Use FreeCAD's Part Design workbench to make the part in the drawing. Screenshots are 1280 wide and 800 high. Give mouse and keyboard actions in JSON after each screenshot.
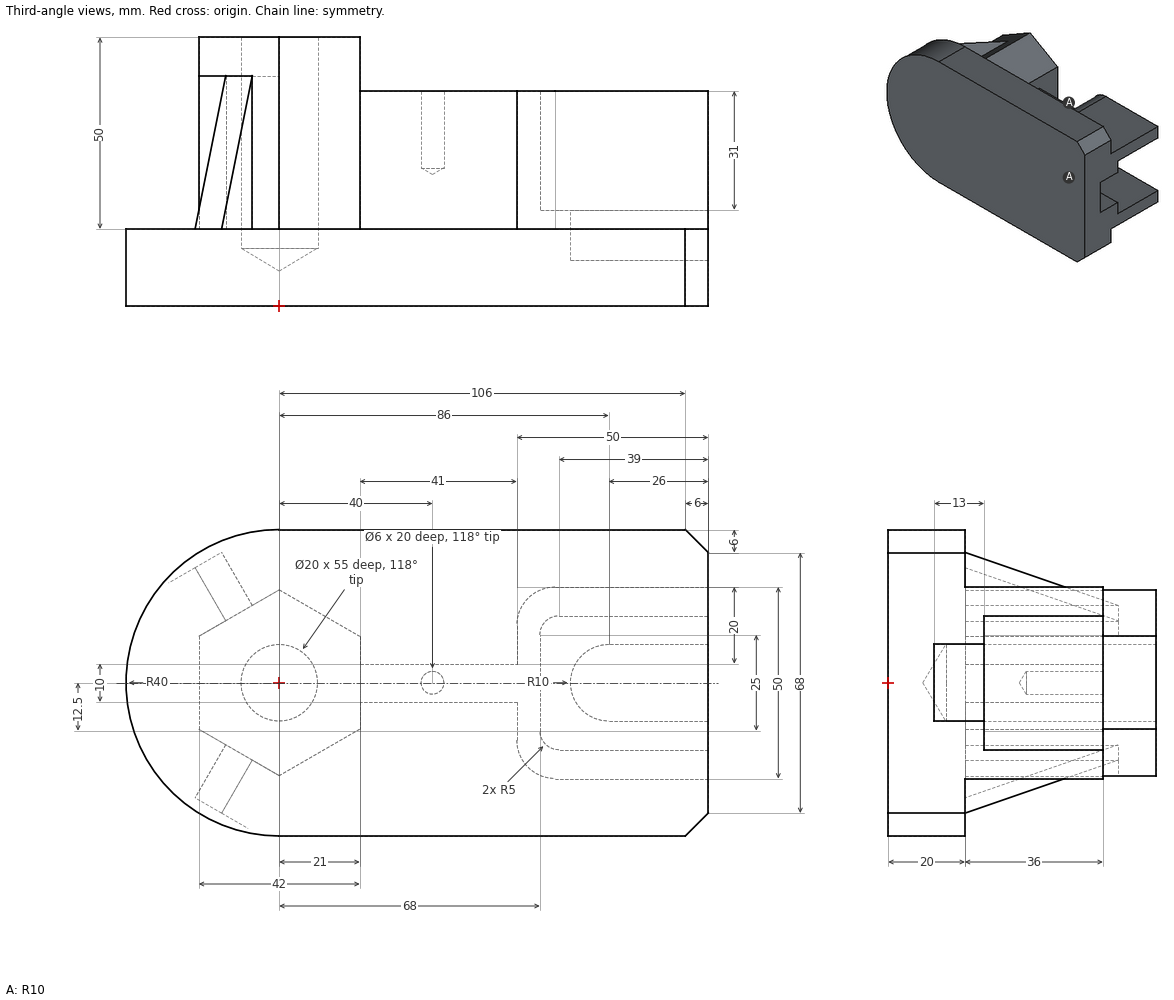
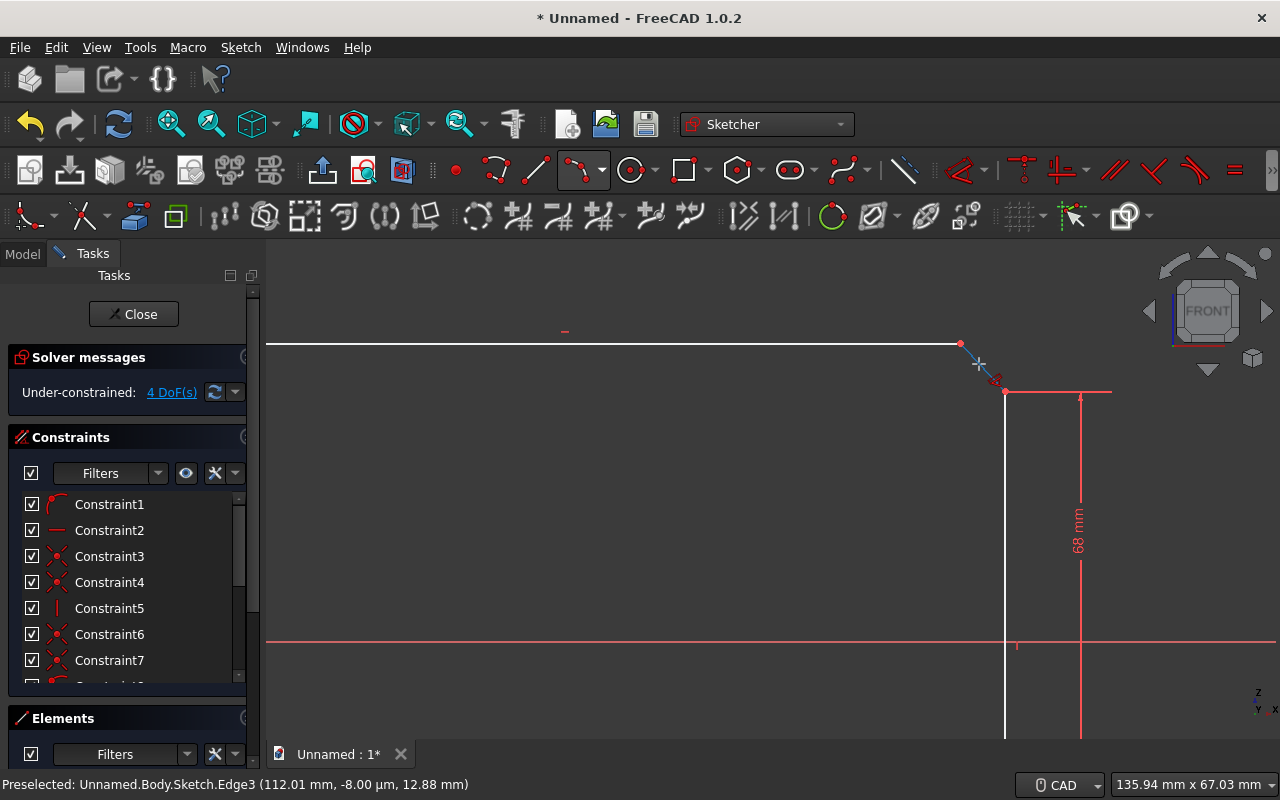
{"action": "left_click", "coordinate": [979, 363]}
{"action": "left_click", "coordinate": [983, 310]}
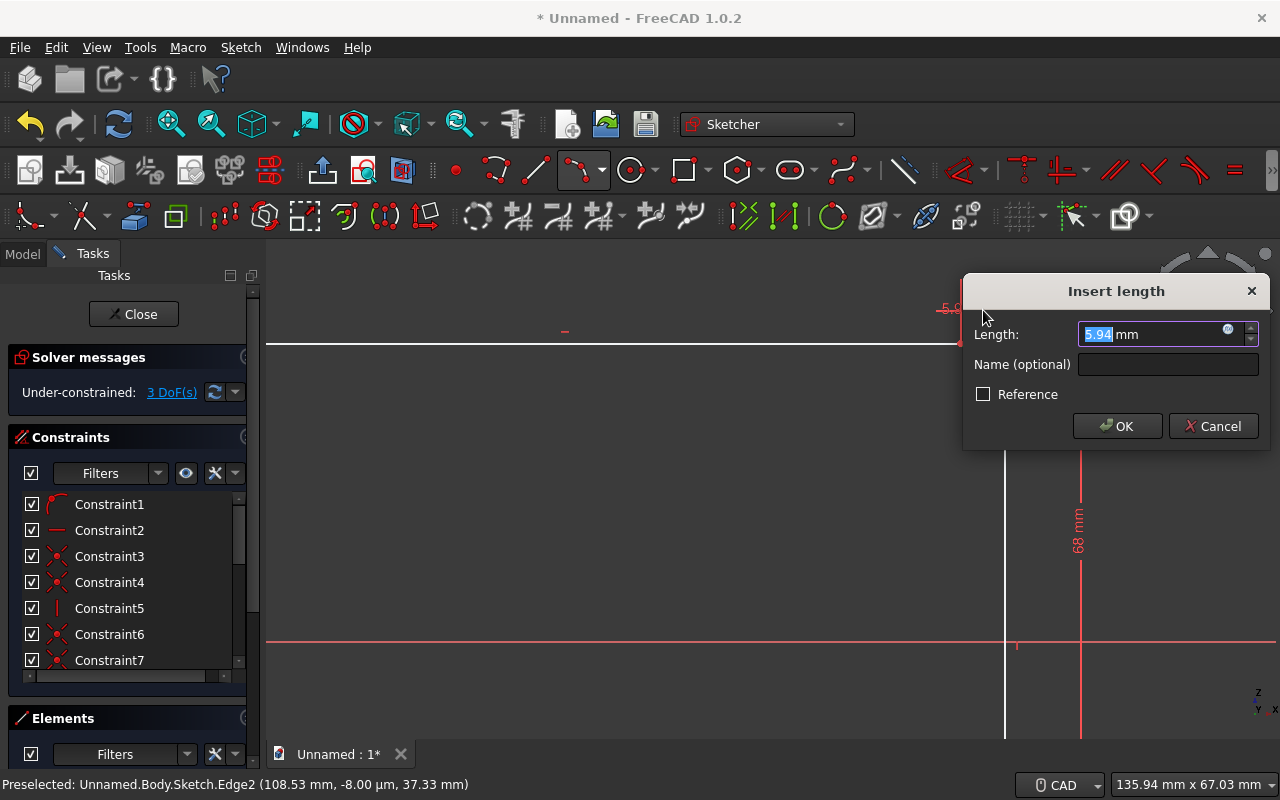
{"action": "type", "text": "6"}
{"action": "key", "text": "Return"}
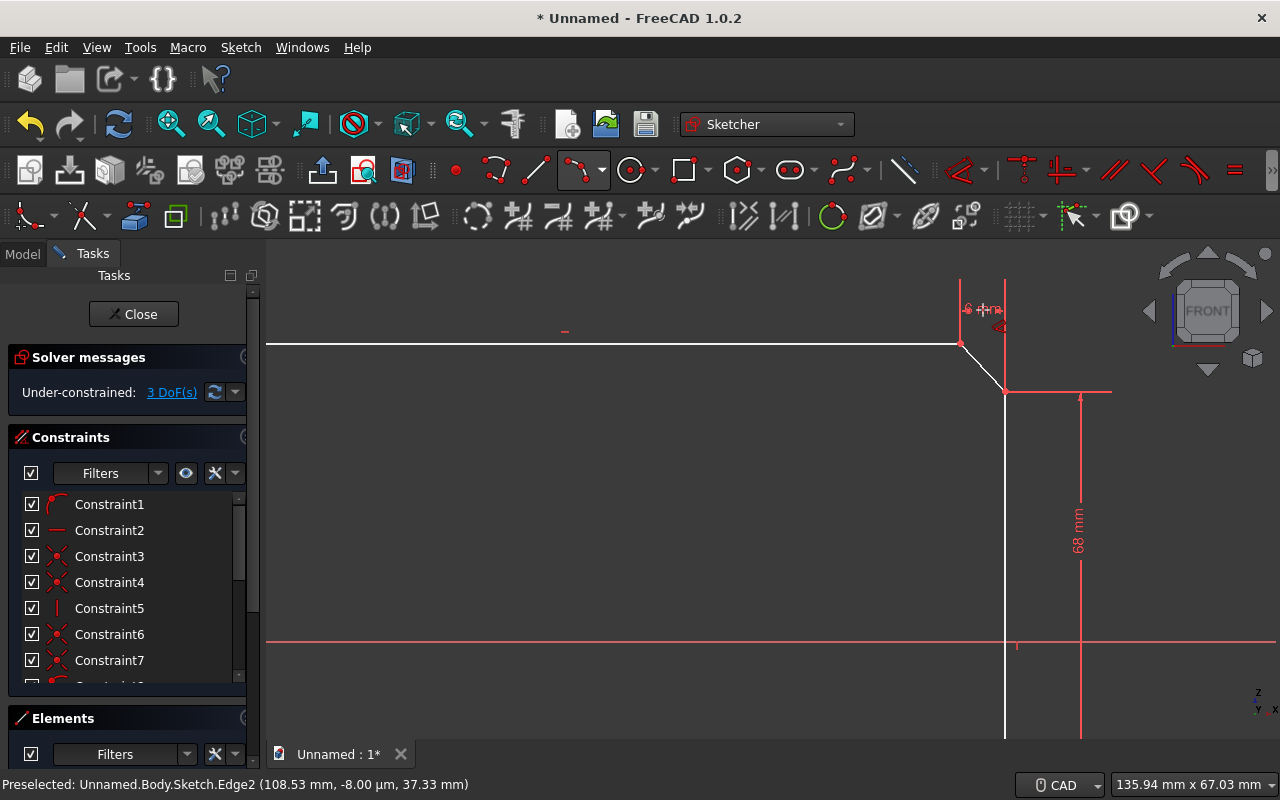
{"action": "left_click", "coordinate": [974, 358]}
{"action": "left_click", "coordinate": [1039, 368]}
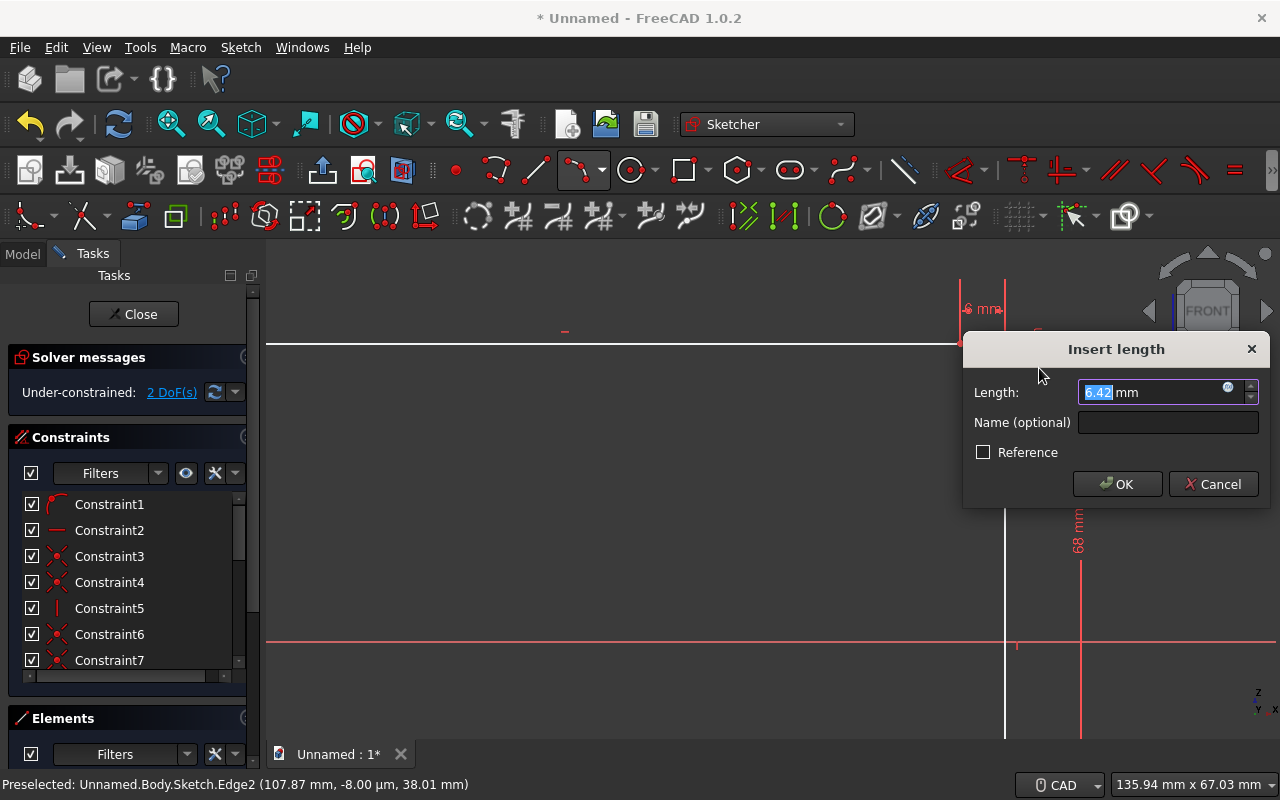
{"action": "type", "text": "6"}
{"action": "key", "text": "Return"}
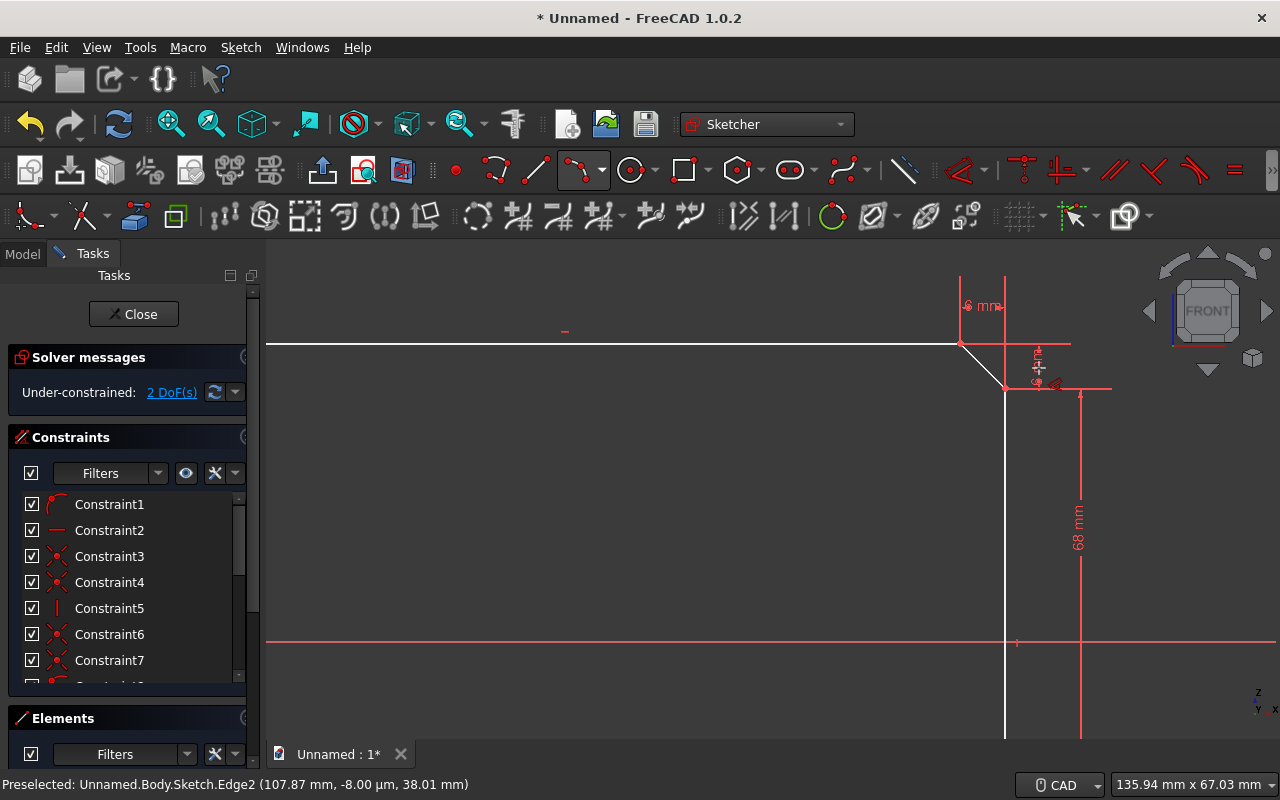
{"action": "scroll", "coordinate": [1028, 303], "scroll_direction": "down", "scroll_amount": 3}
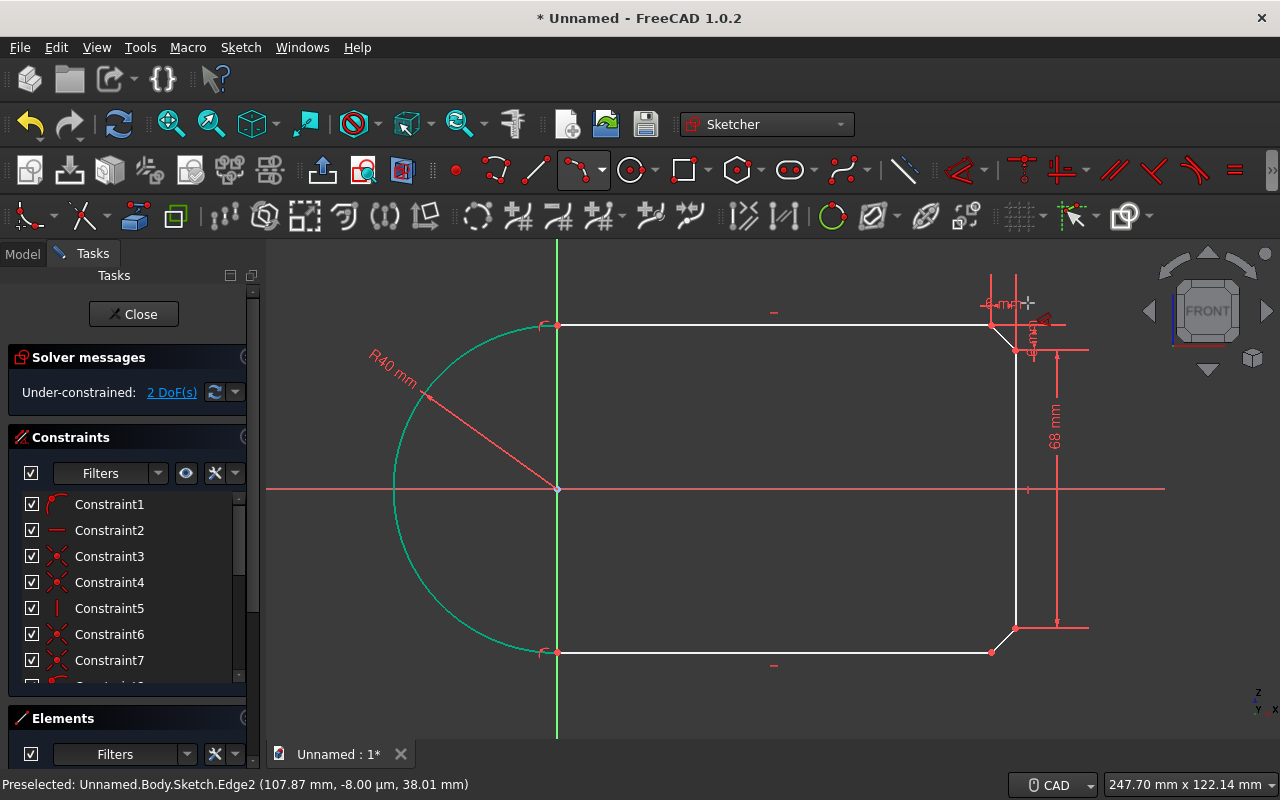
{"action": "scroll", "coordinate": [1008, 636], "scroll_direction": "up", "scroll_amount": 3}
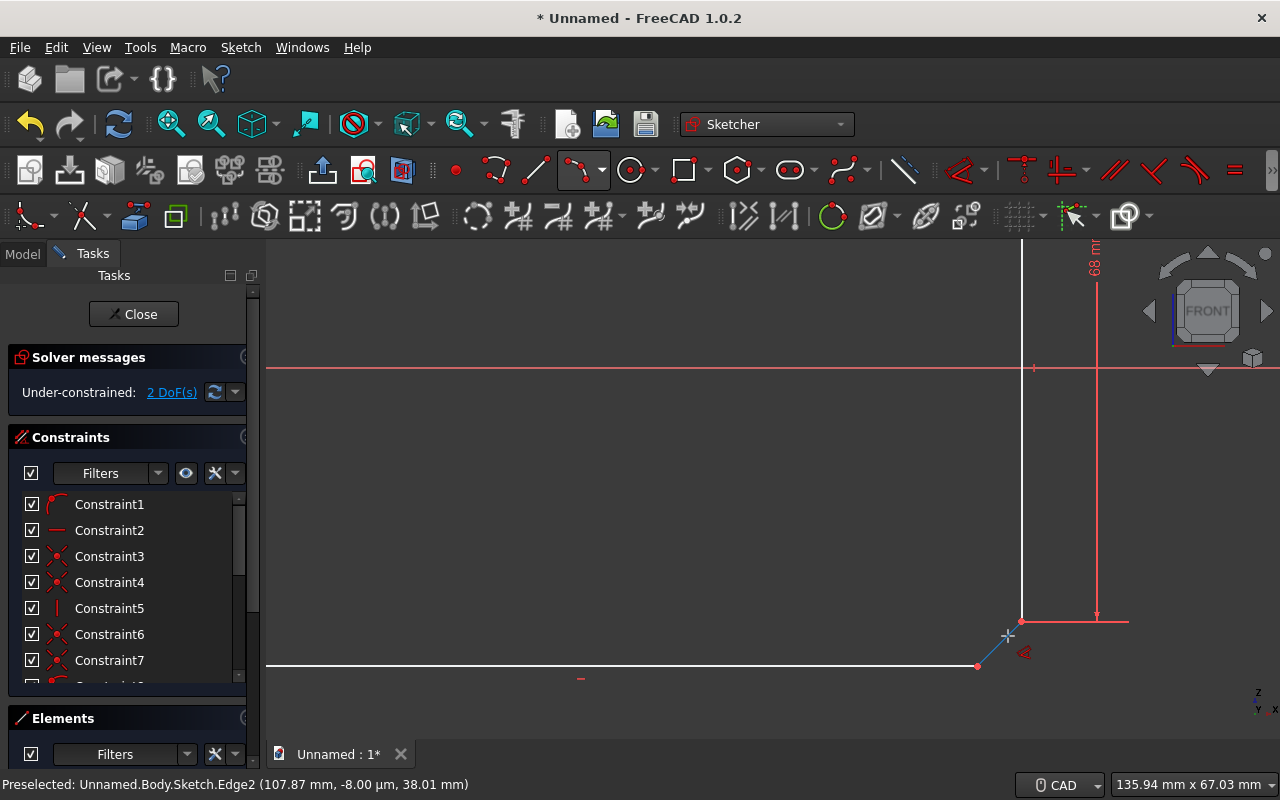
{"action": "left_click", "coordinate": [1008, 635]}
{"action": "left_click", "coordinate": [999, 700]}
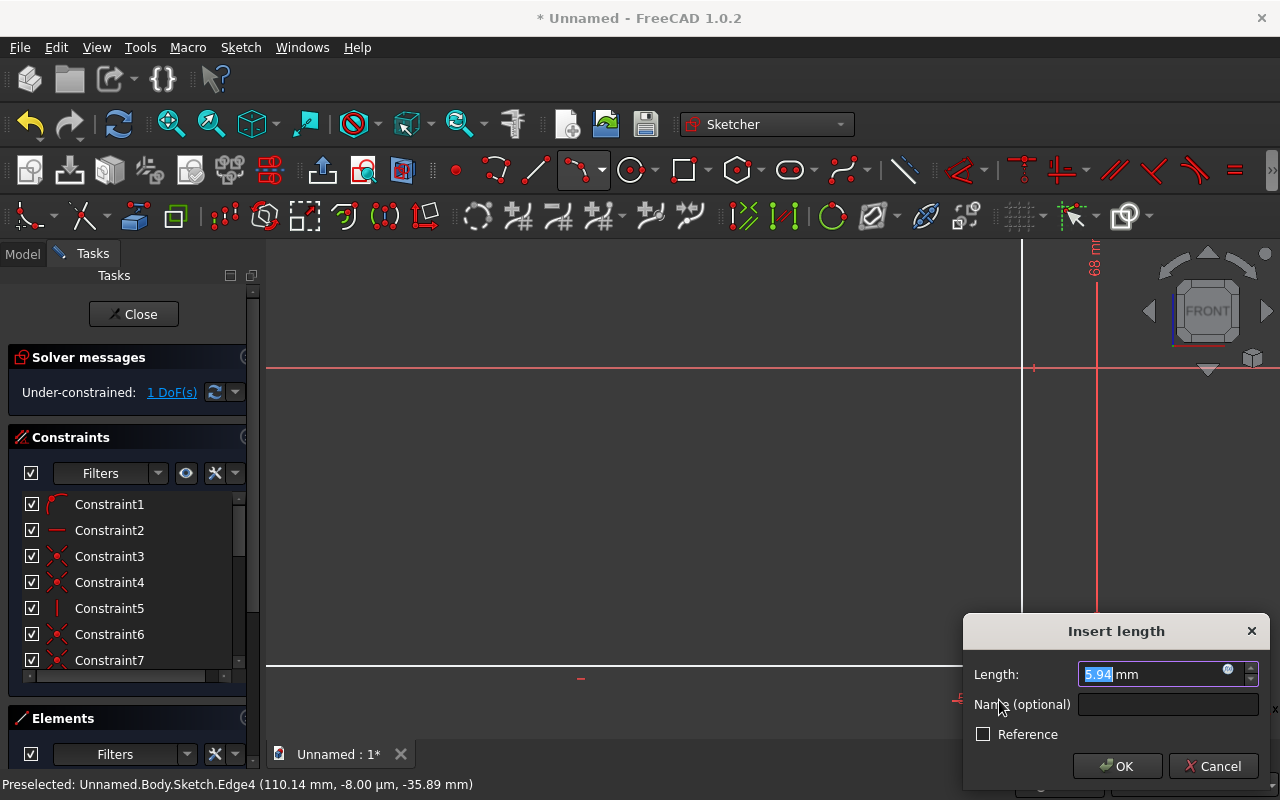
{"action": "type", "text": "6"}
{"action": "key", "text": "Return"}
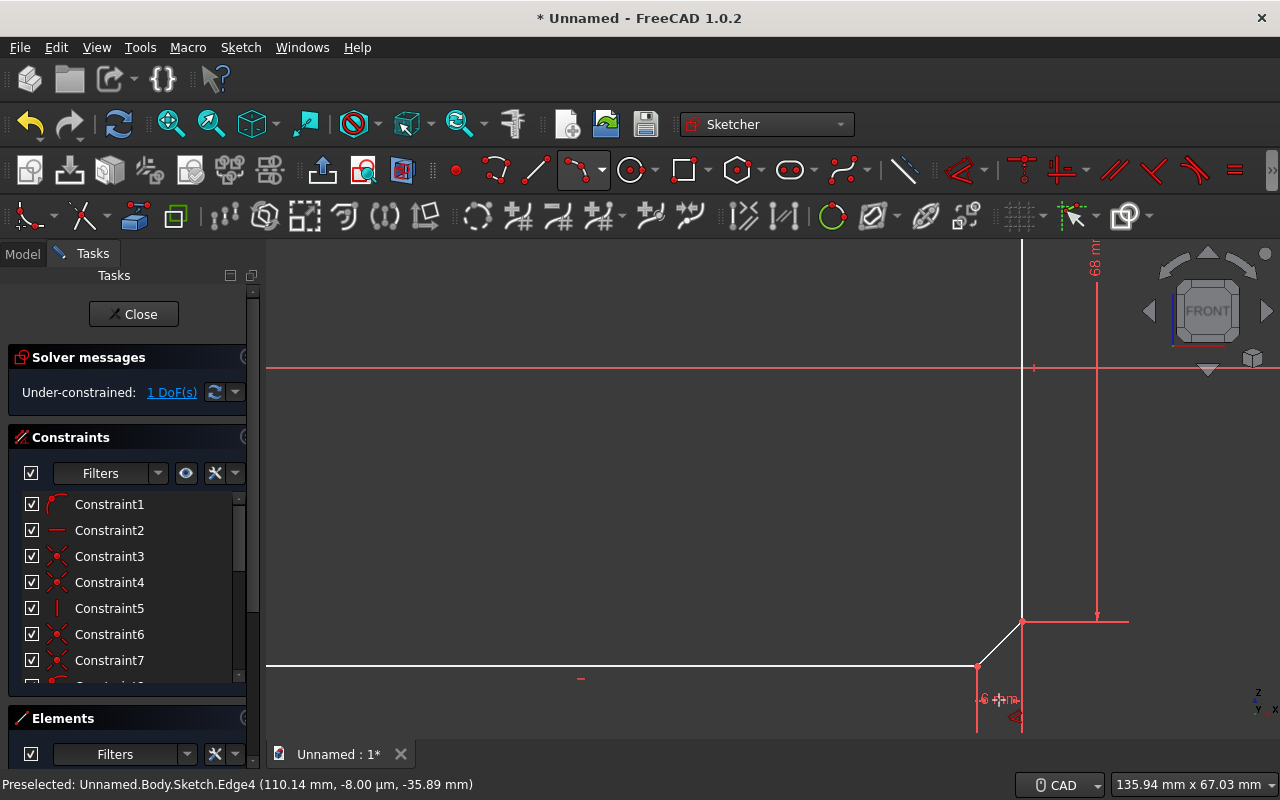
{"action": "scroll", "coordinate": [1008, 636], "scroll_direction": "down", "scroll_amount": 3}